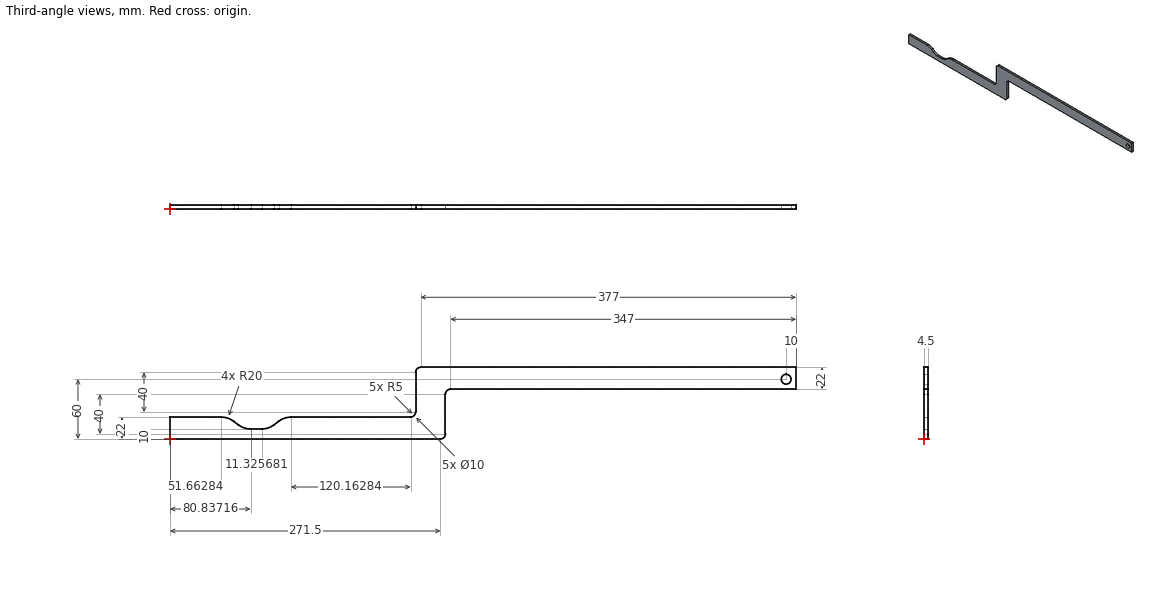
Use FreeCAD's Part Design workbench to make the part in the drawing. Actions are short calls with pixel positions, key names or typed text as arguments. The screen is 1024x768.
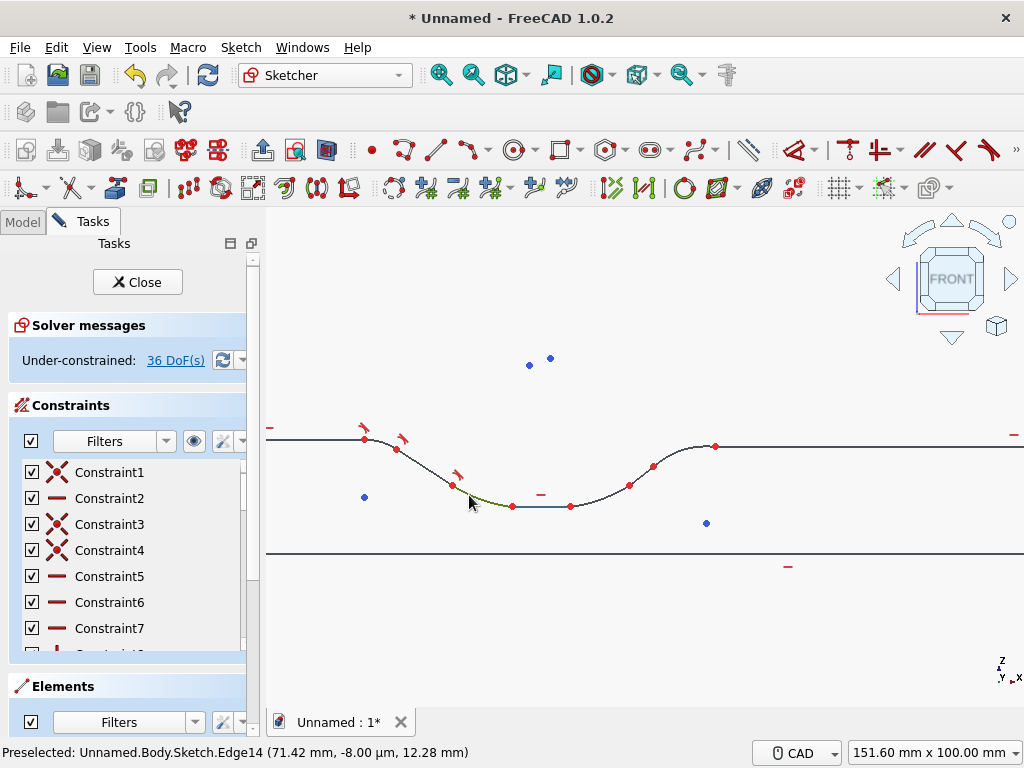
key(t)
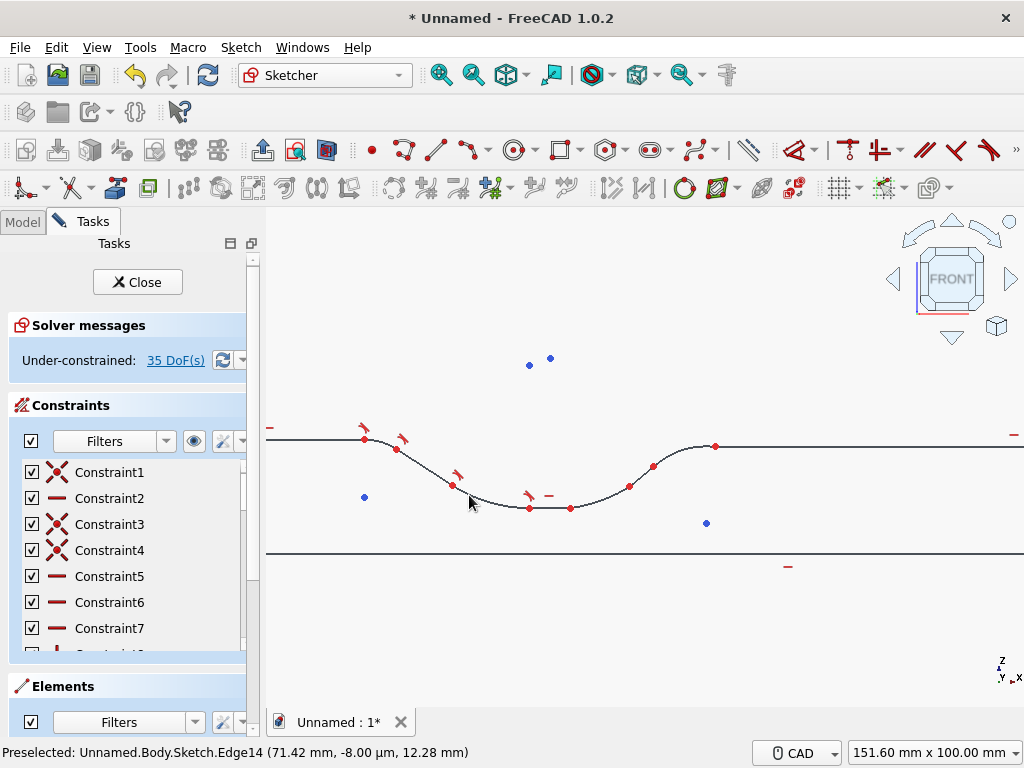
click(542, 508)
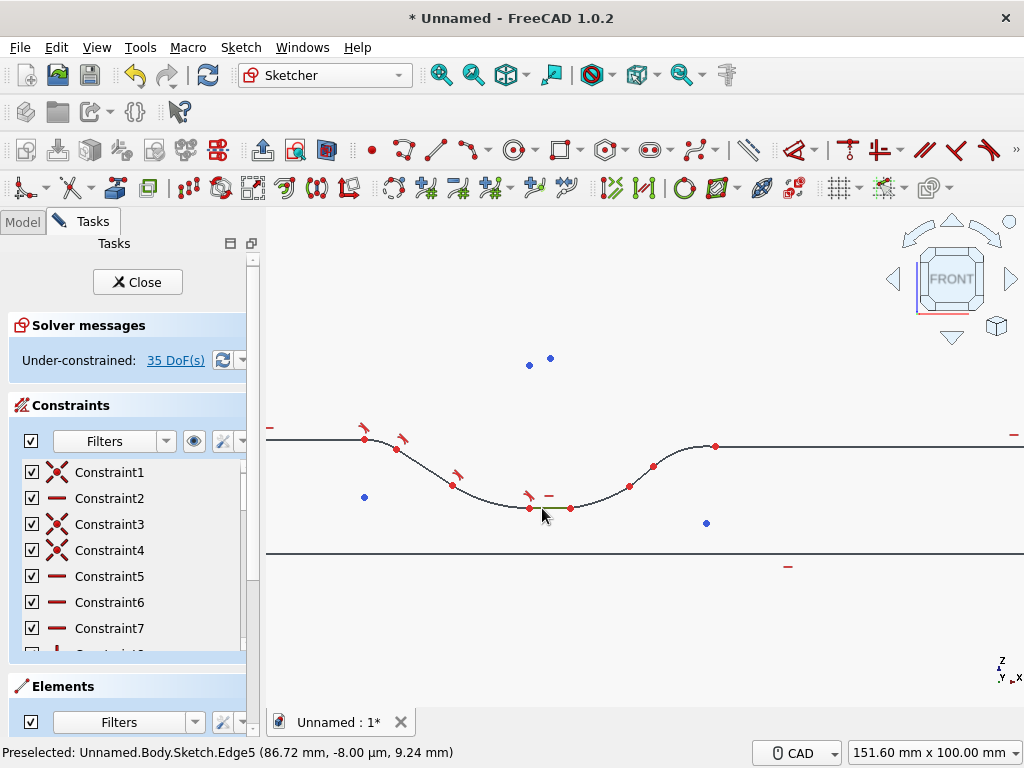
click(589, 504)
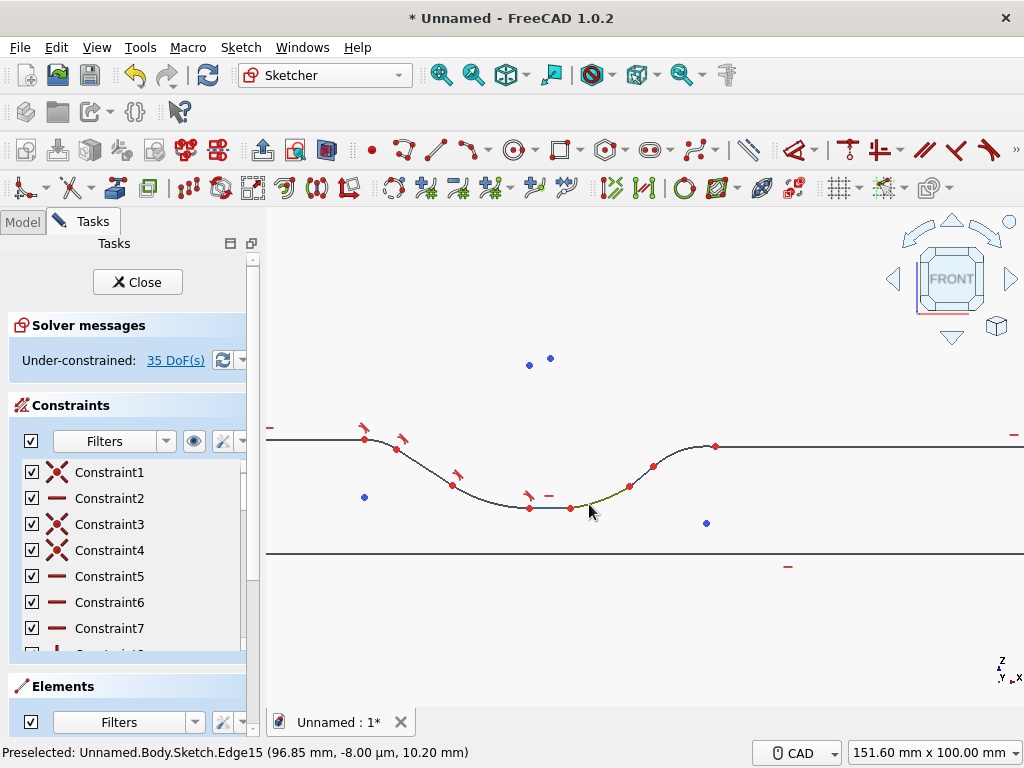
key(t)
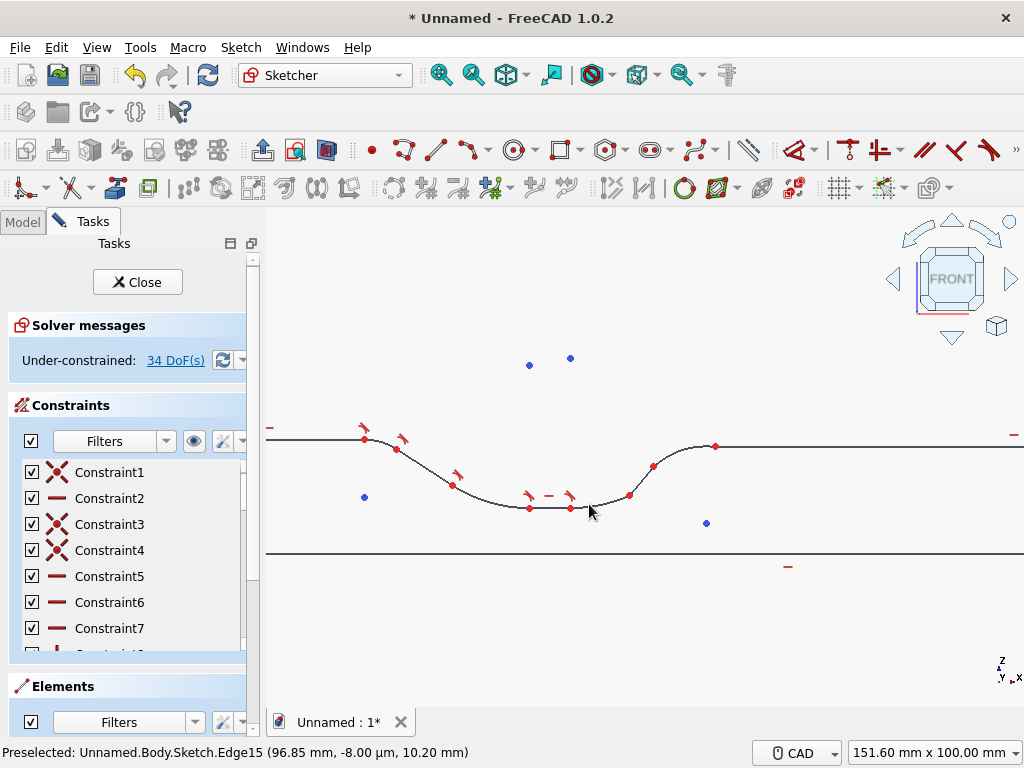
scroll(637, 487, up, 2)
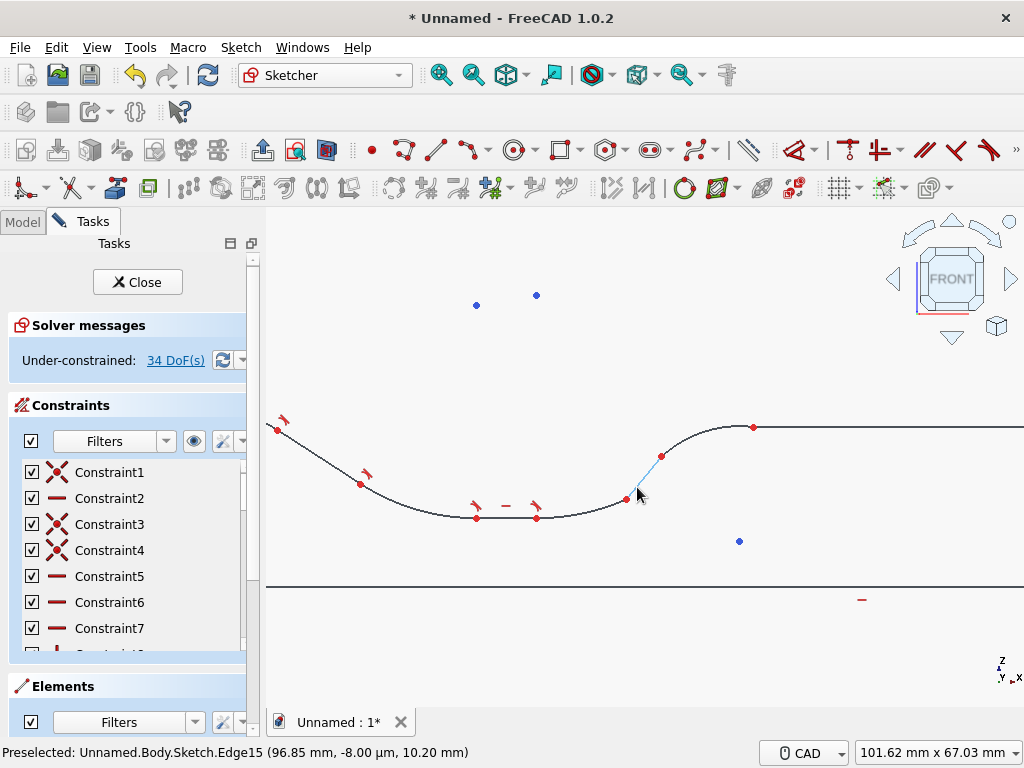
click(637, 487)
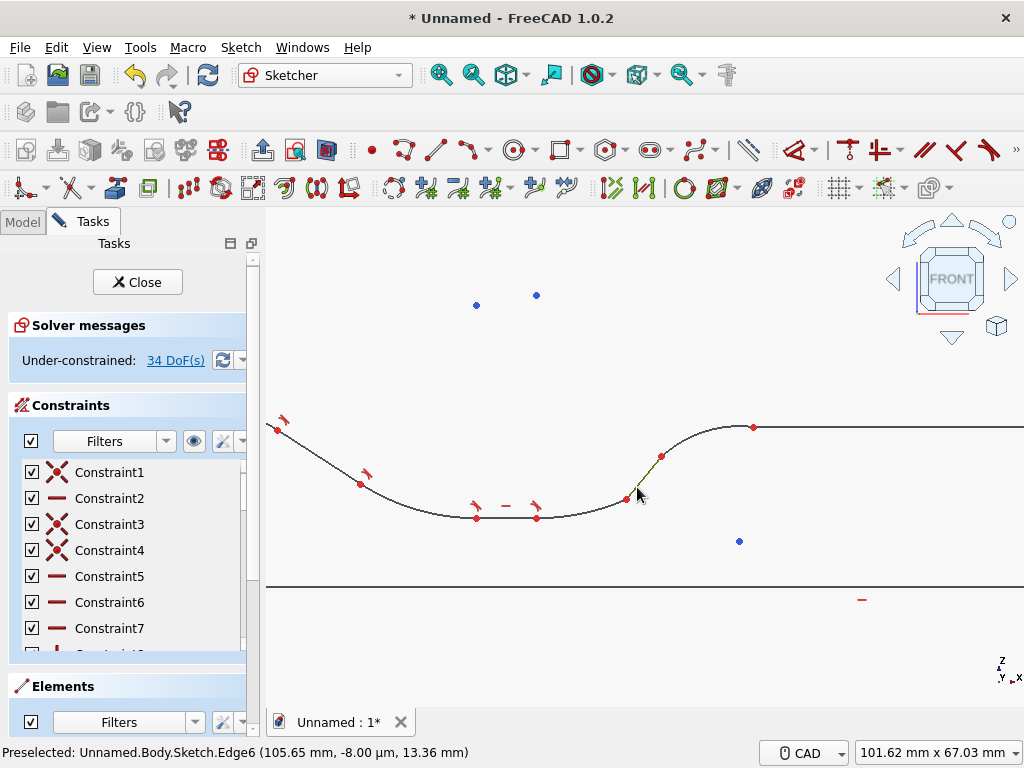
click(564, 516)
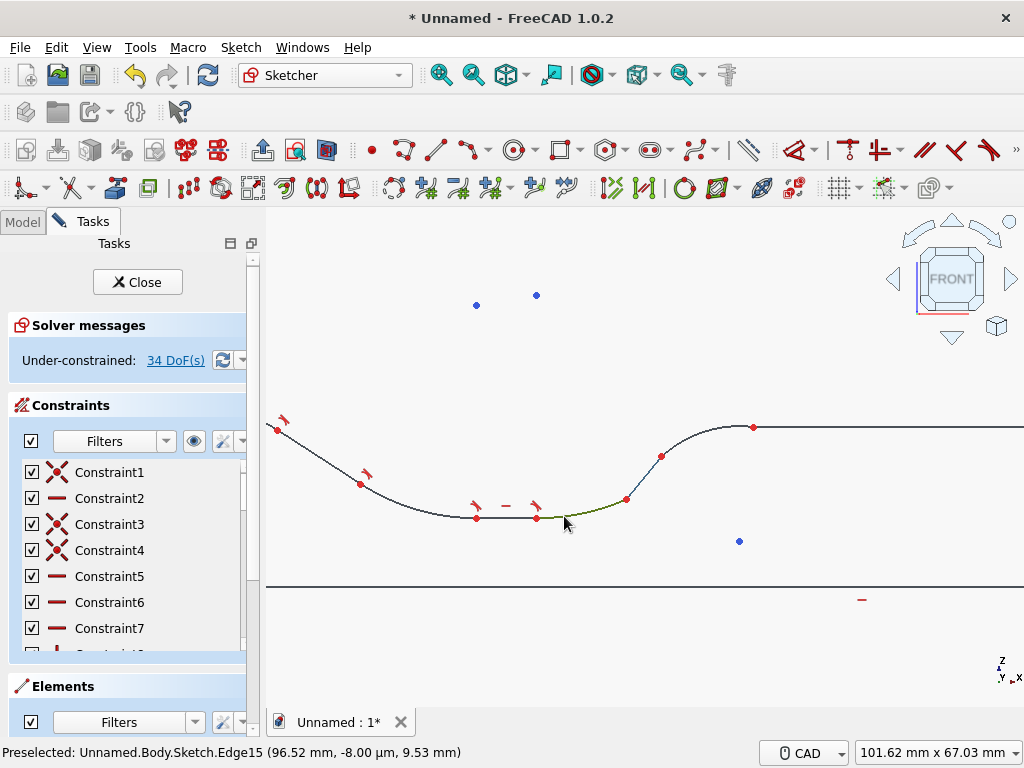
click(990, 150)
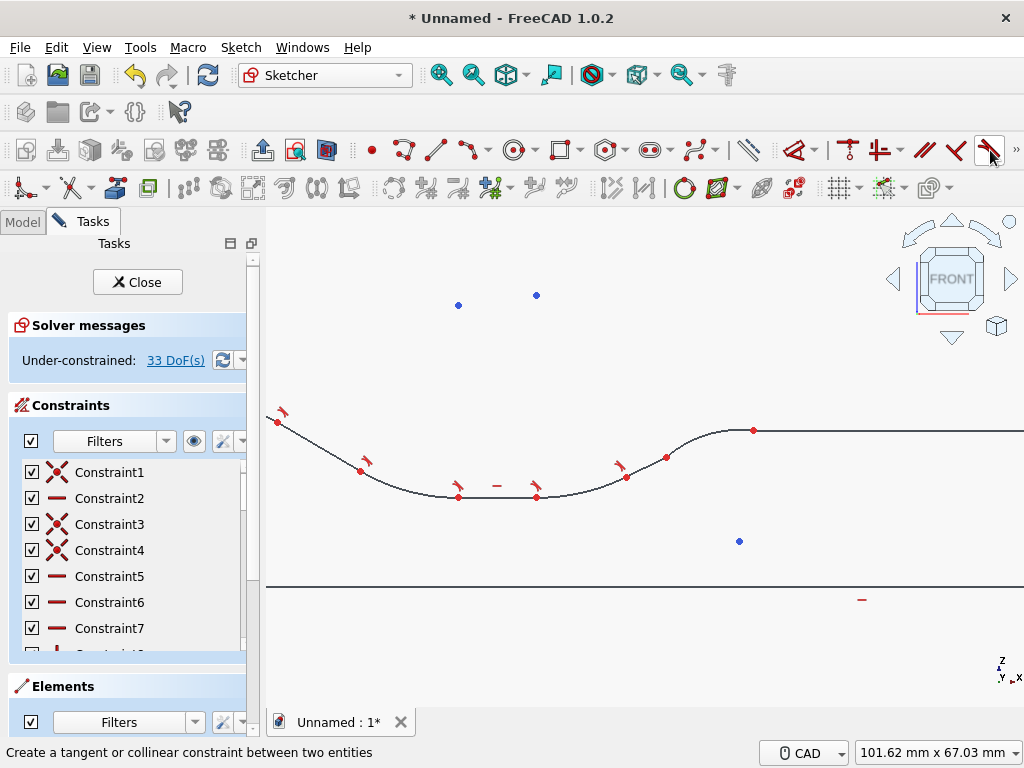
click(638, 471)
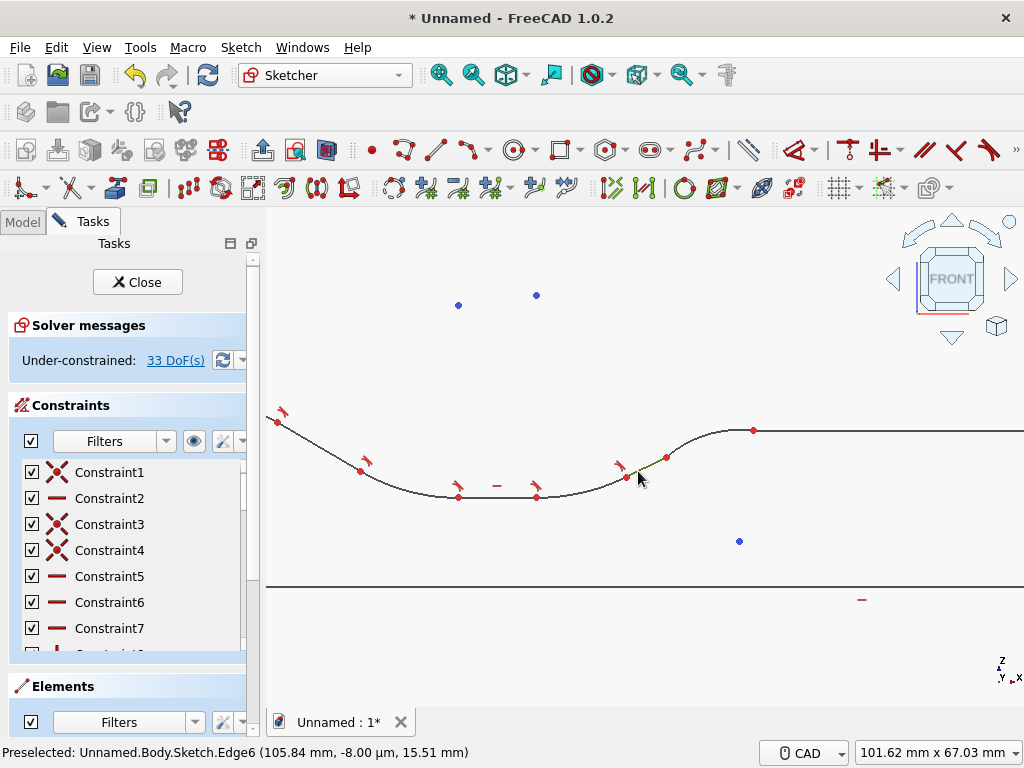
click(726, 431)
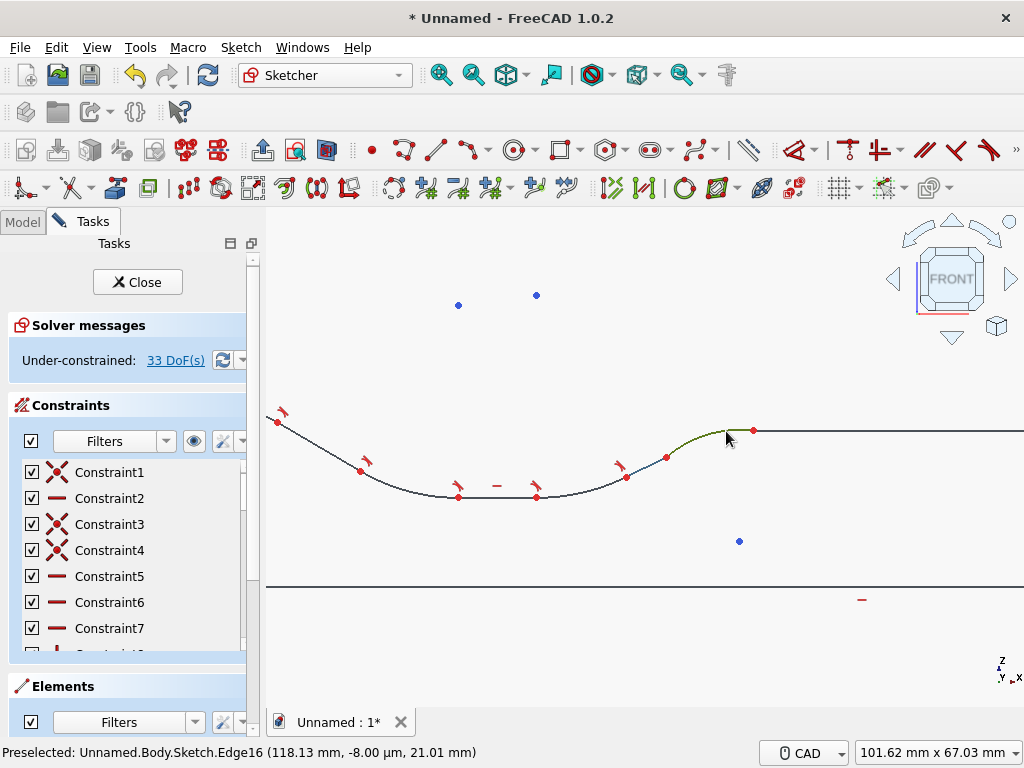
key(t)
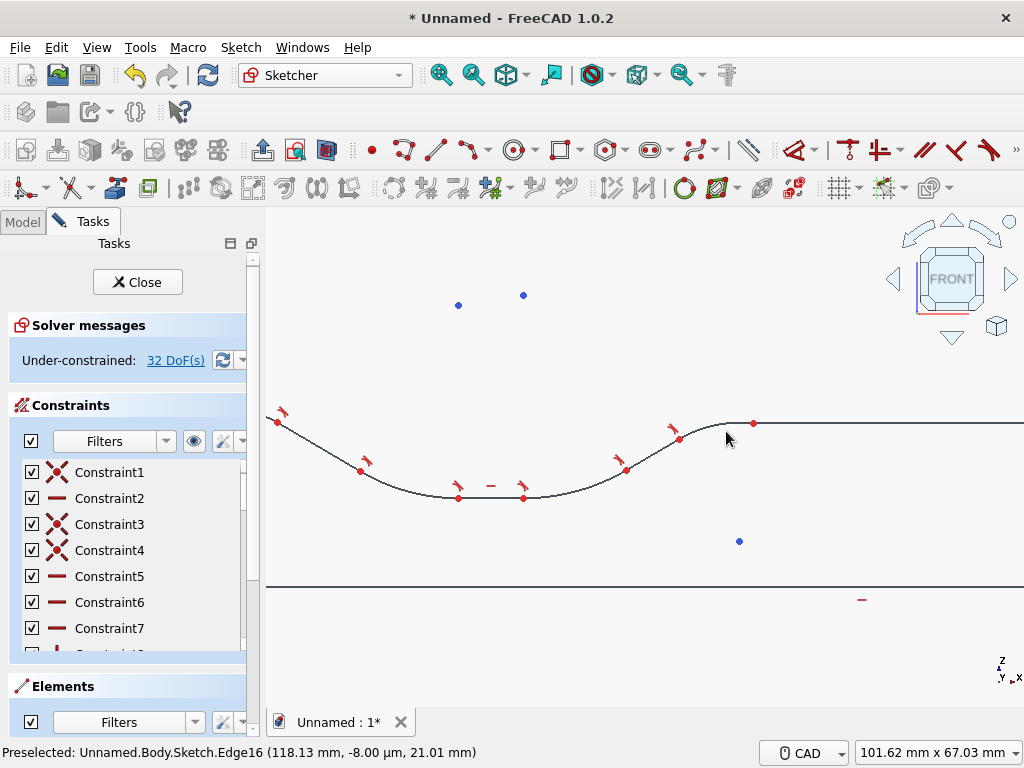
scroll(415, 471, down, 12)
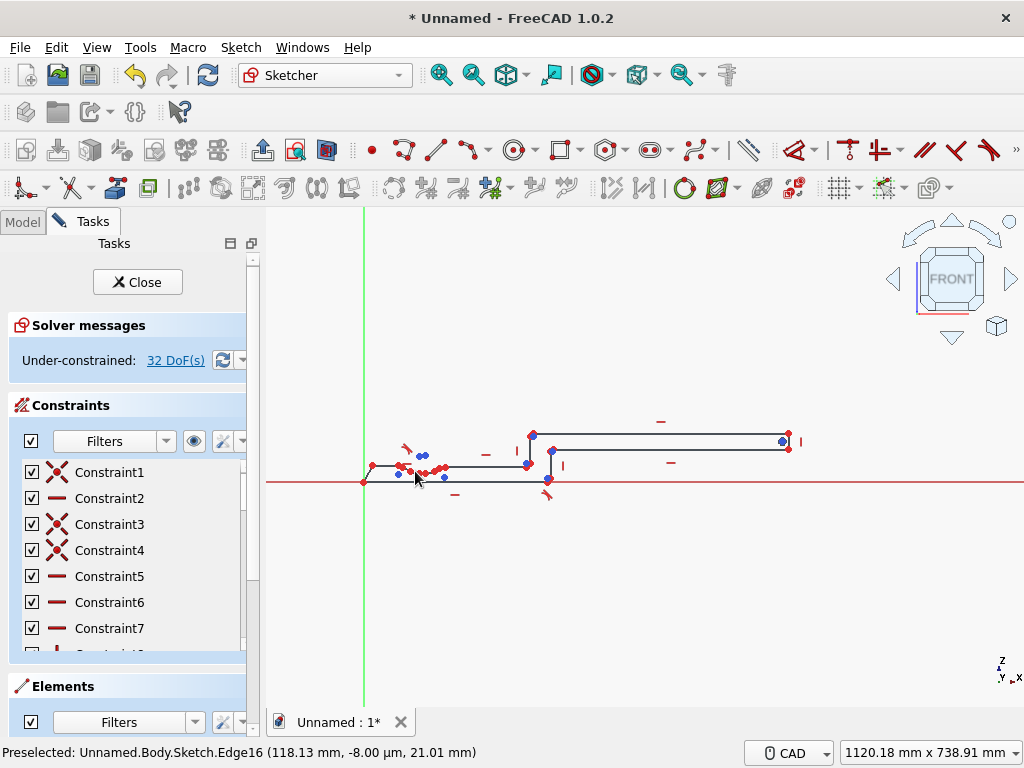
click(470, 467)